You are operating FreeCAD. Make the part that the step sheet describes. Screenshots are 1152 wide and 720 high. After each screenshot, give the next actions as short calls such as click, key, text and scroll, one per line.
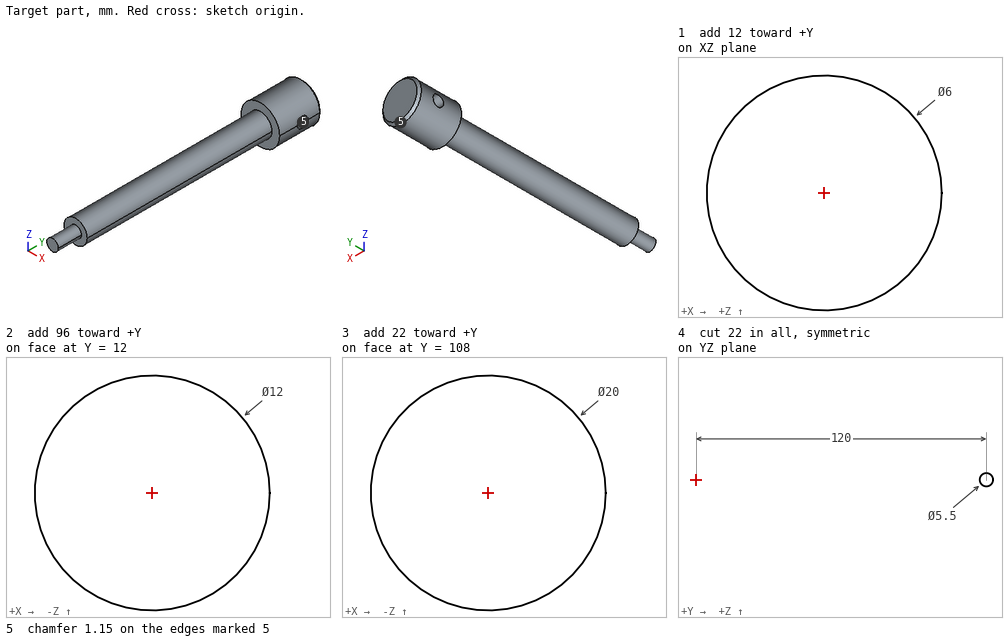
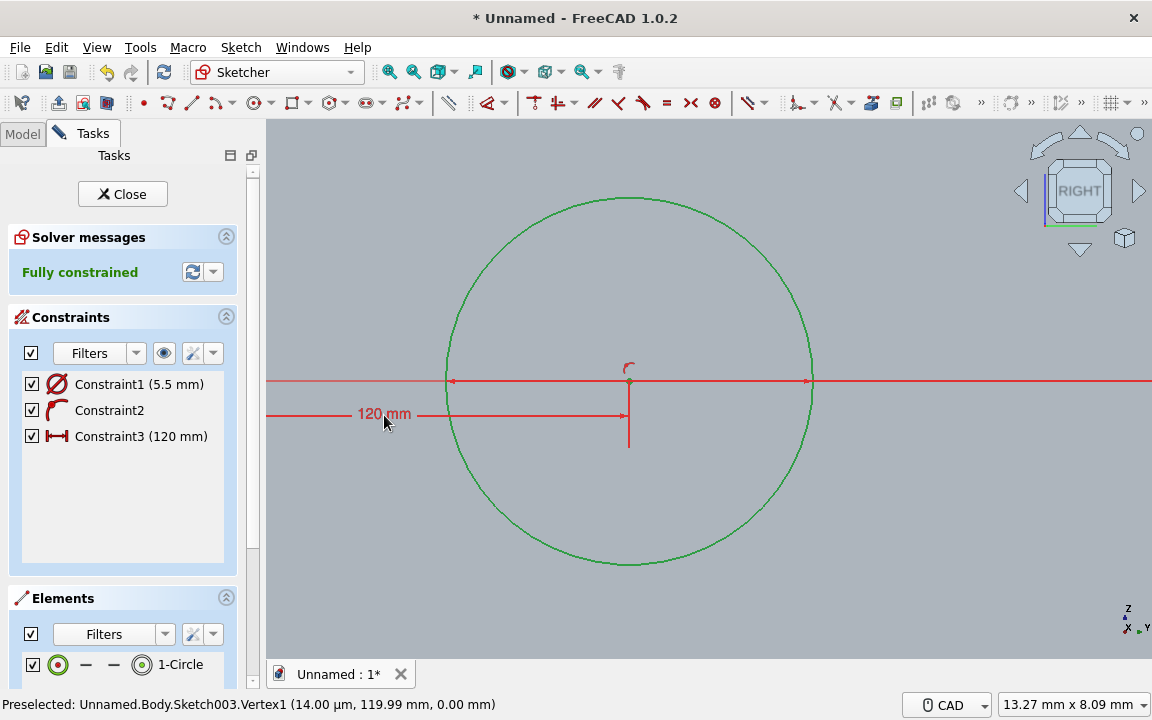
click(123, 194)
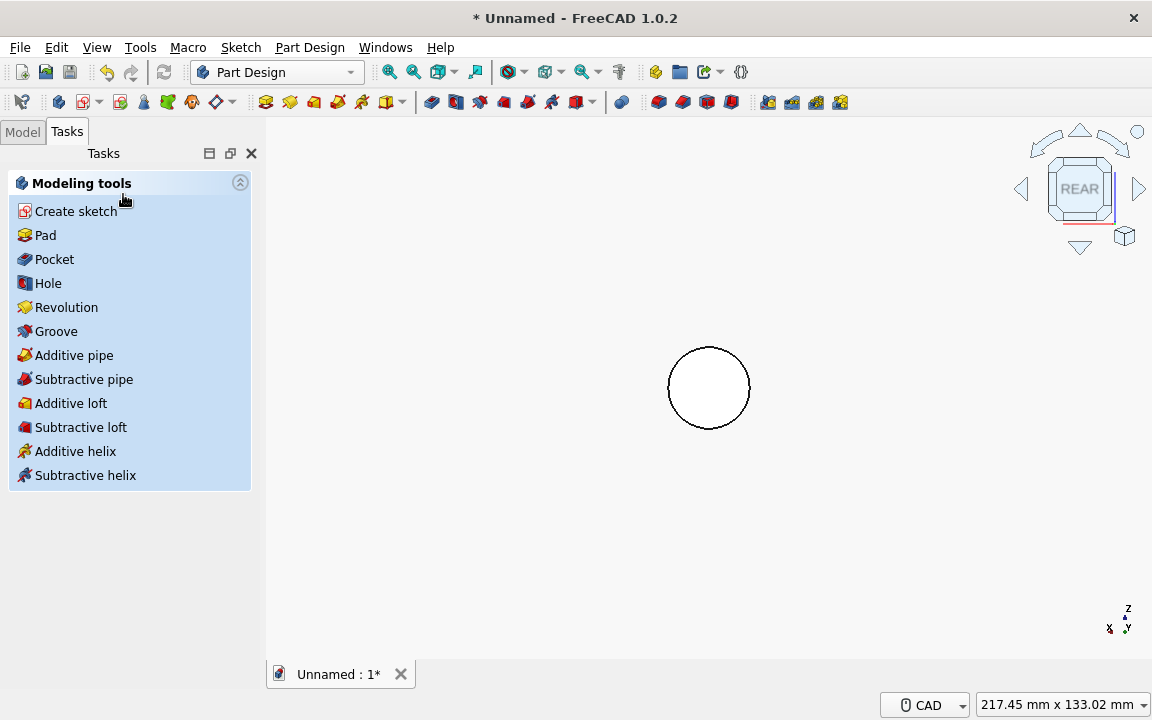
click(432, 102)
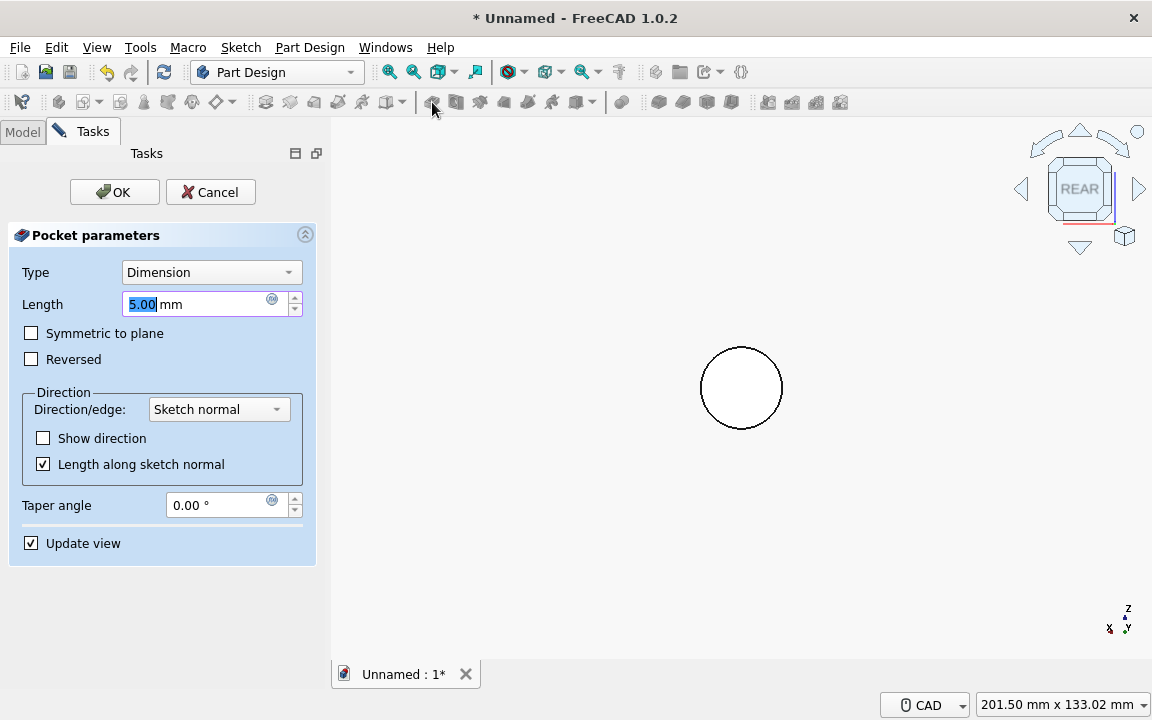
text(22)
key(Tab)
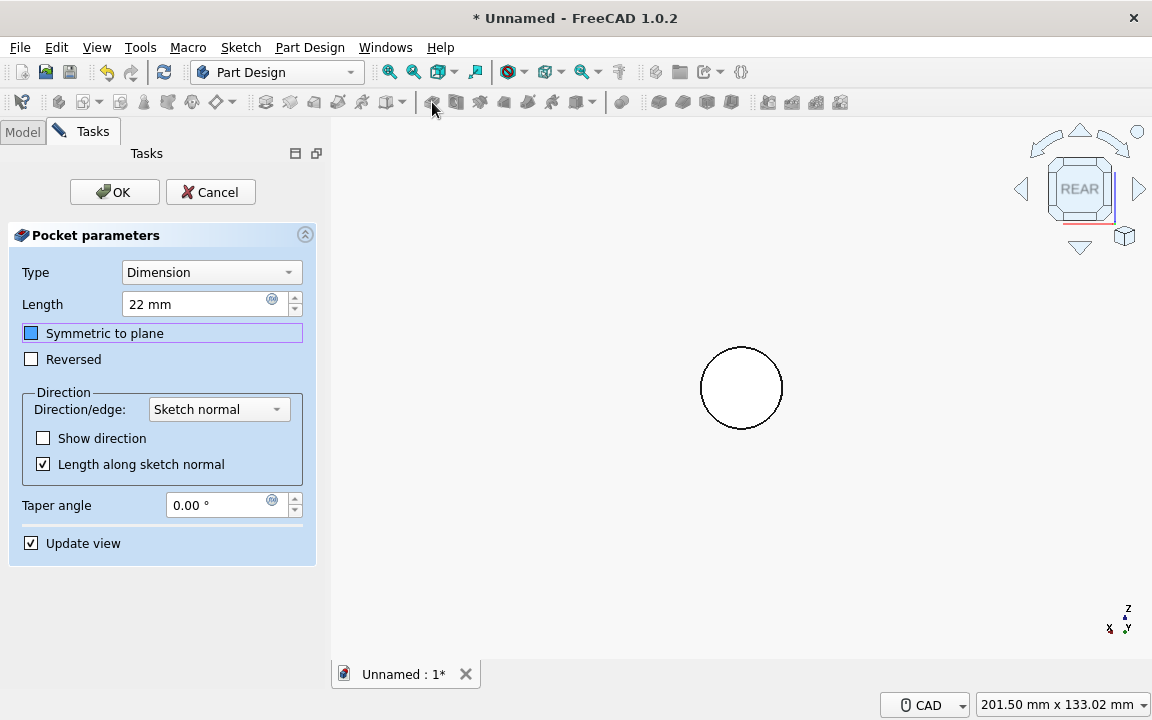
click(30, 333)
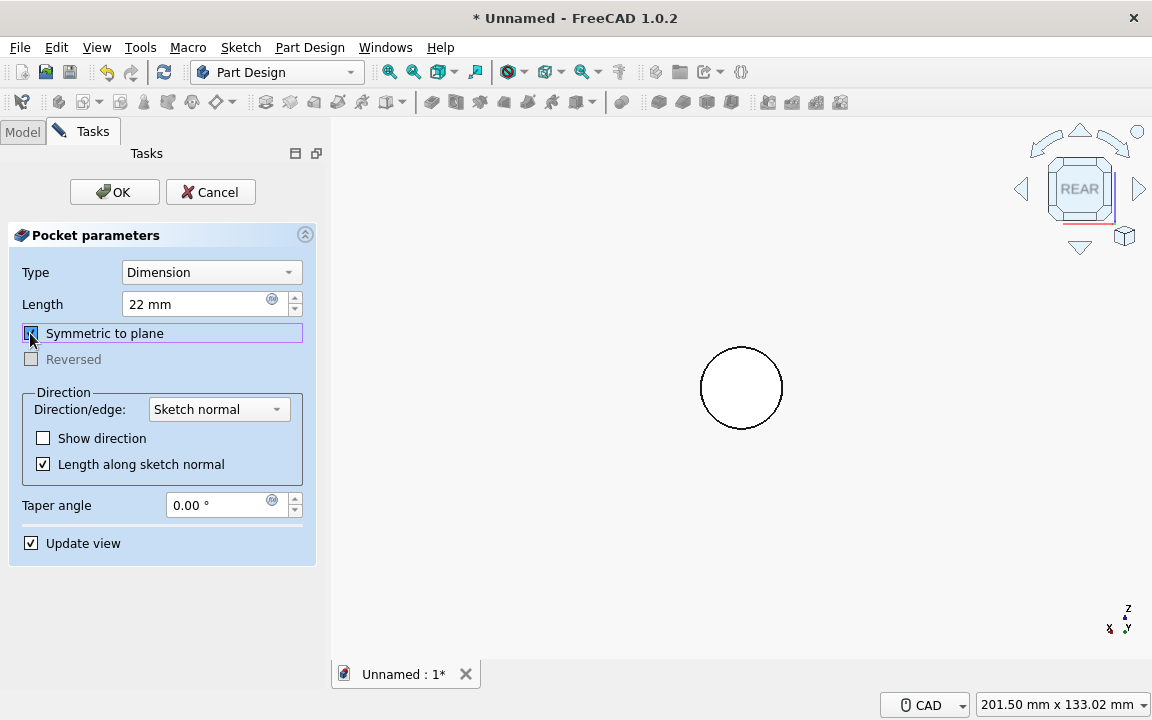
click(115, 192)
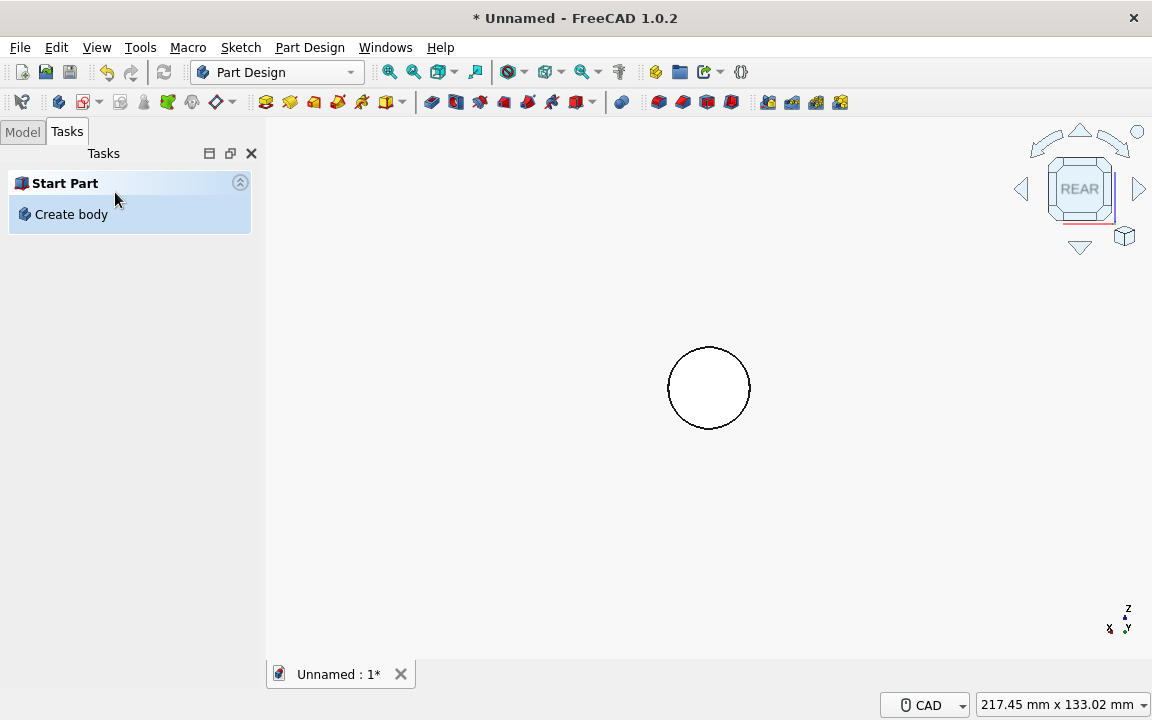
click(390, 72)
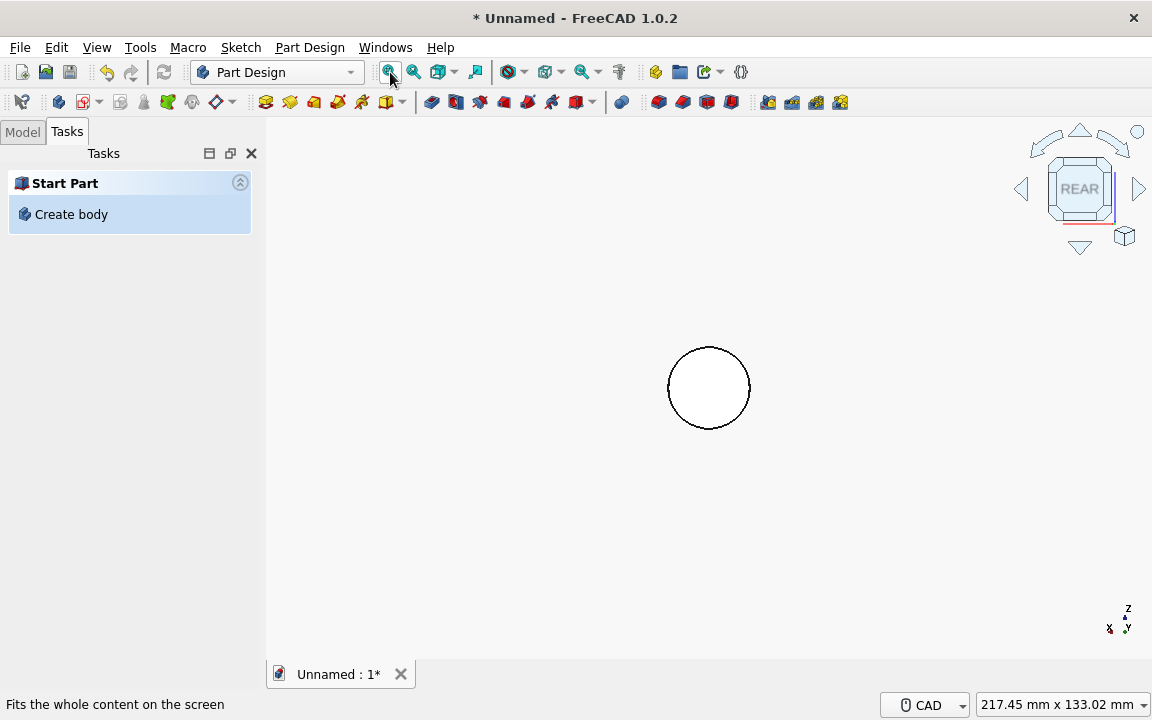
click(750, 387)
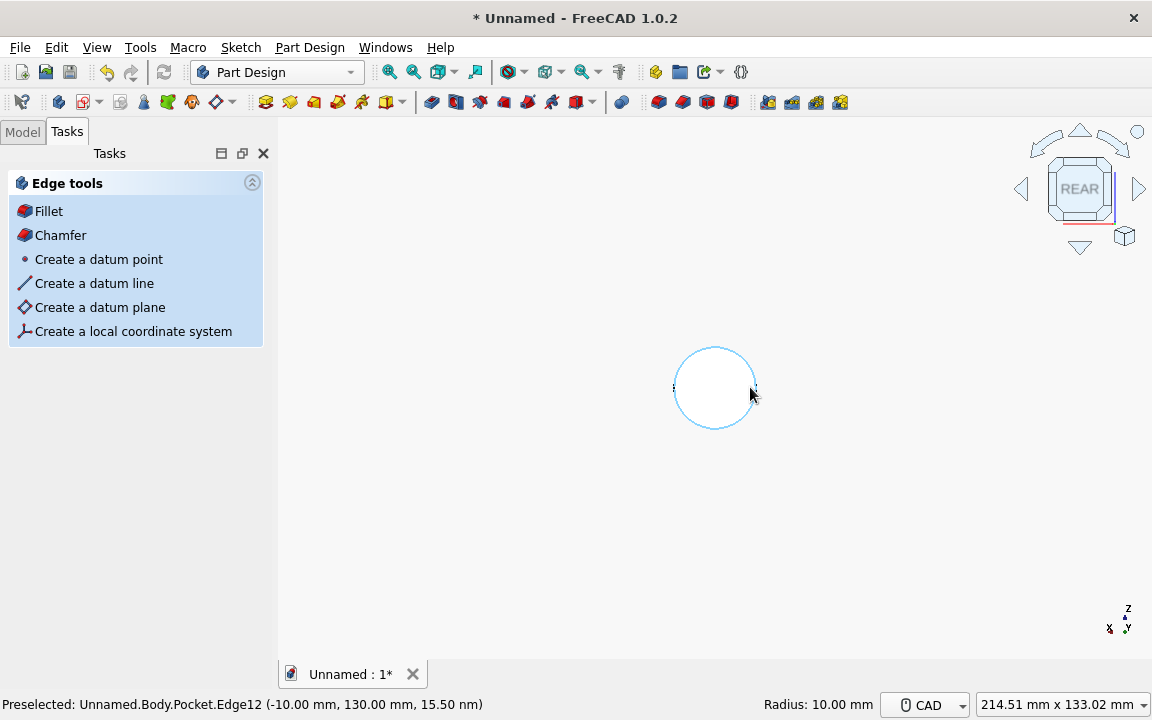
click(684, 102)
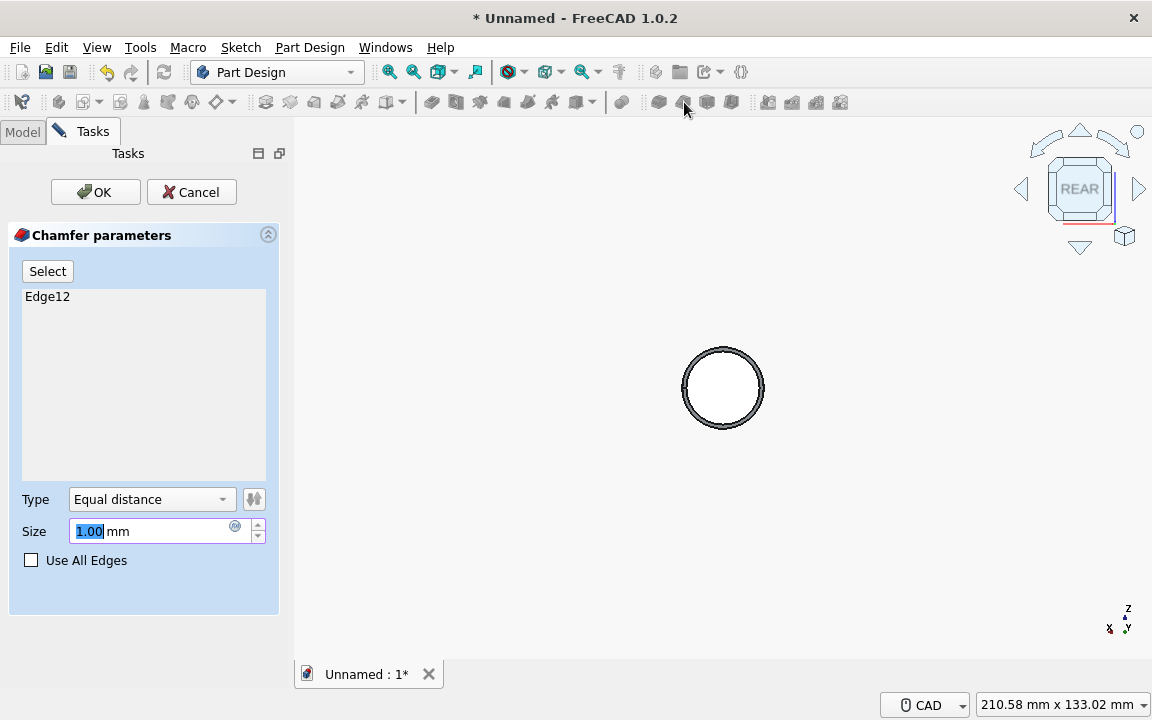
text(1.15)
key(Tab)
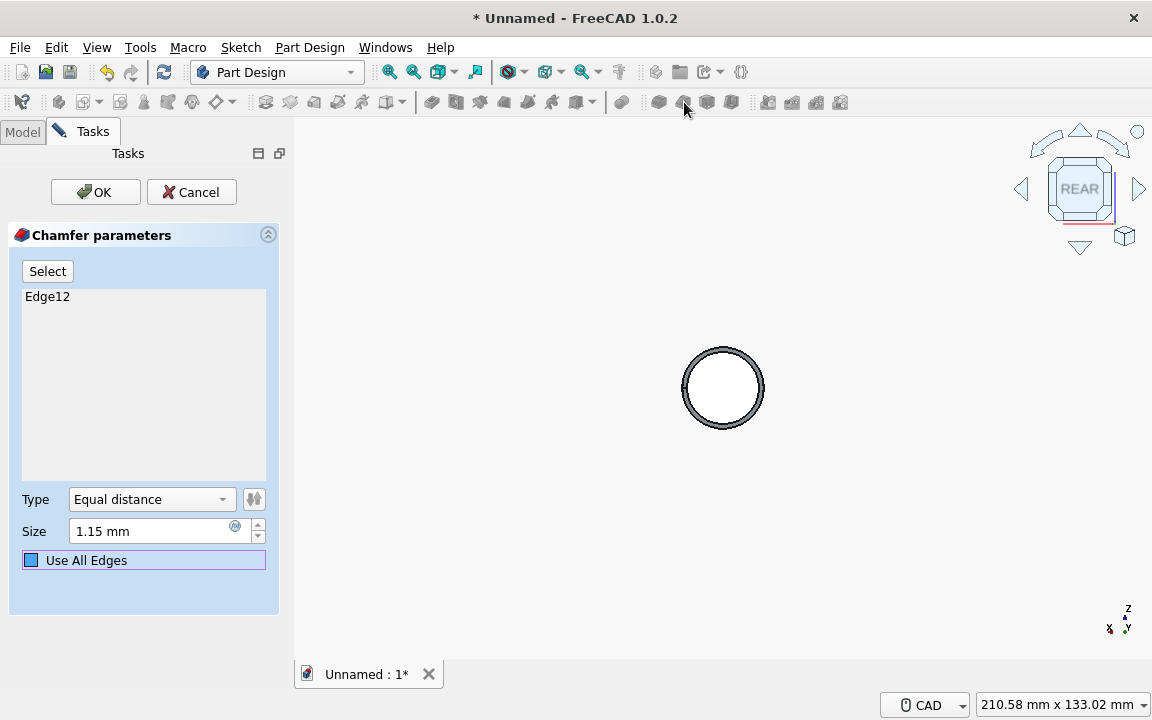
click(96, 192)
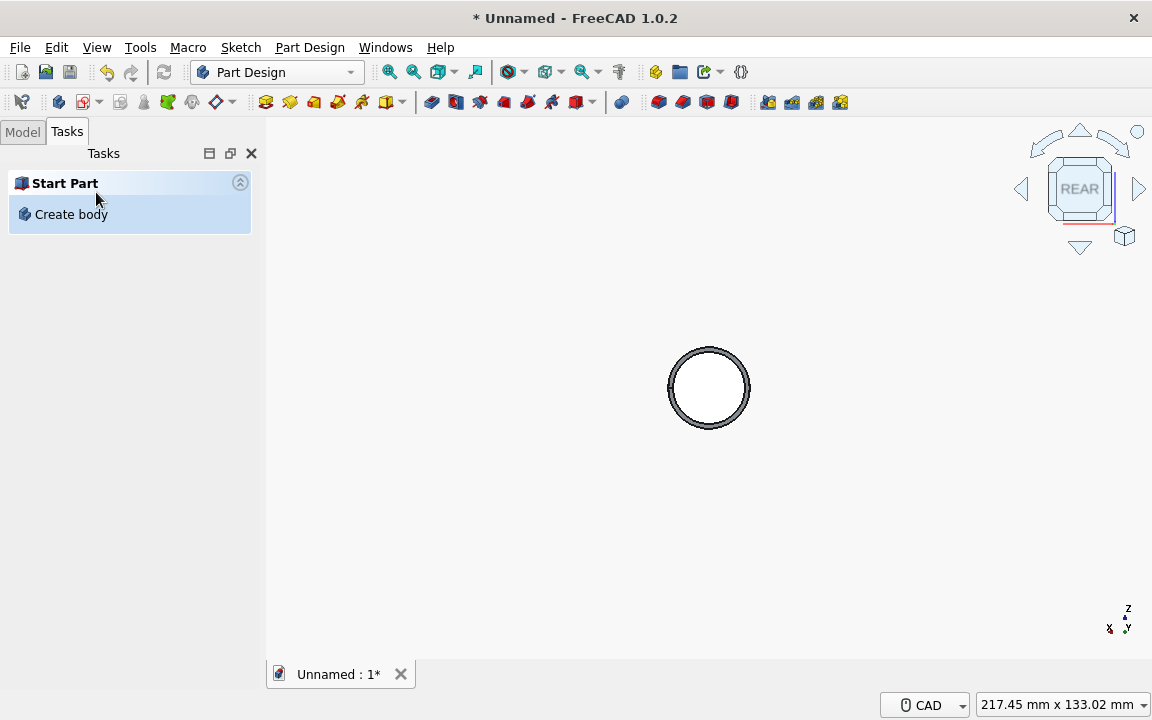
key(0)